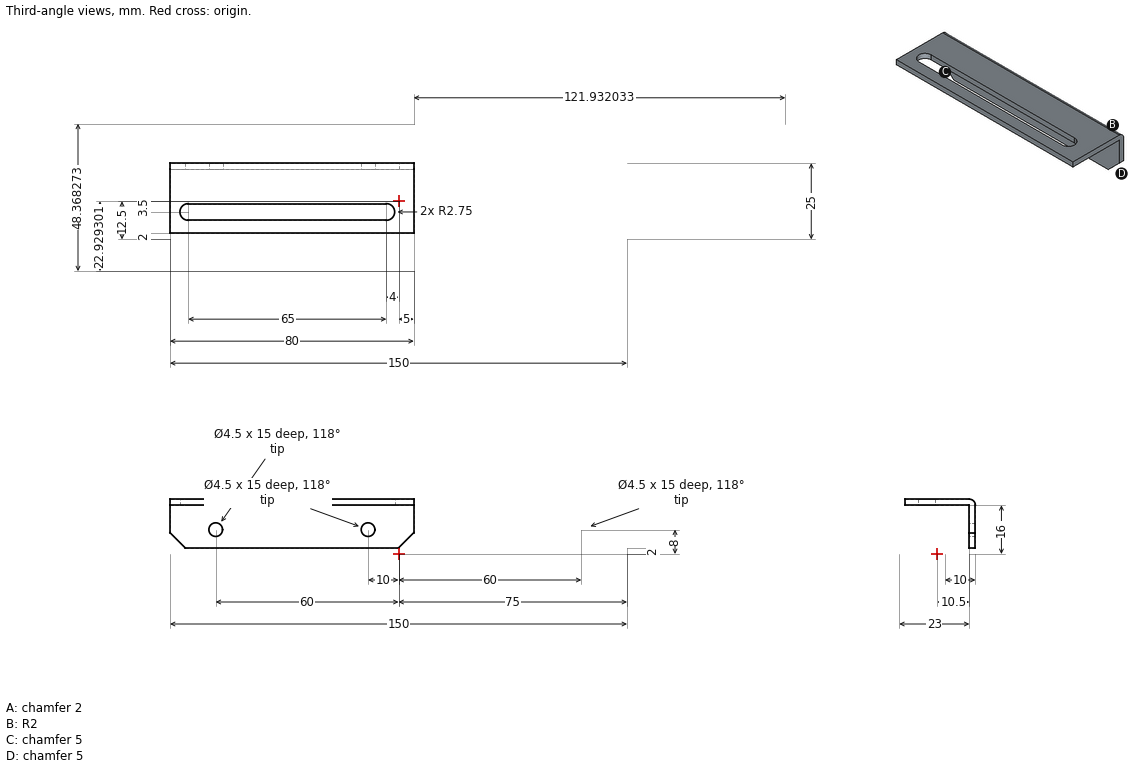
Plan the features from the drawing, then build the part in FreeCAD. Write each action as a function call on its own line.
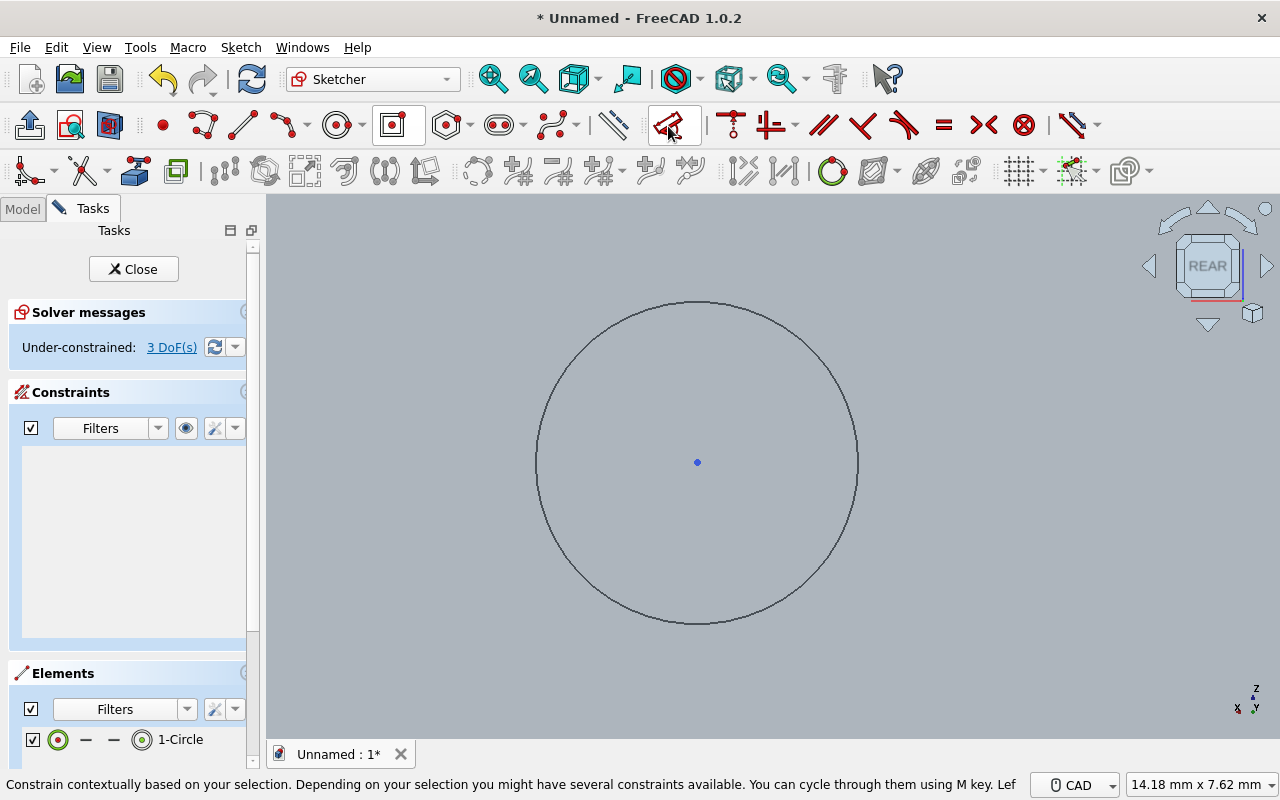
click(811, 349)
click(834, 326)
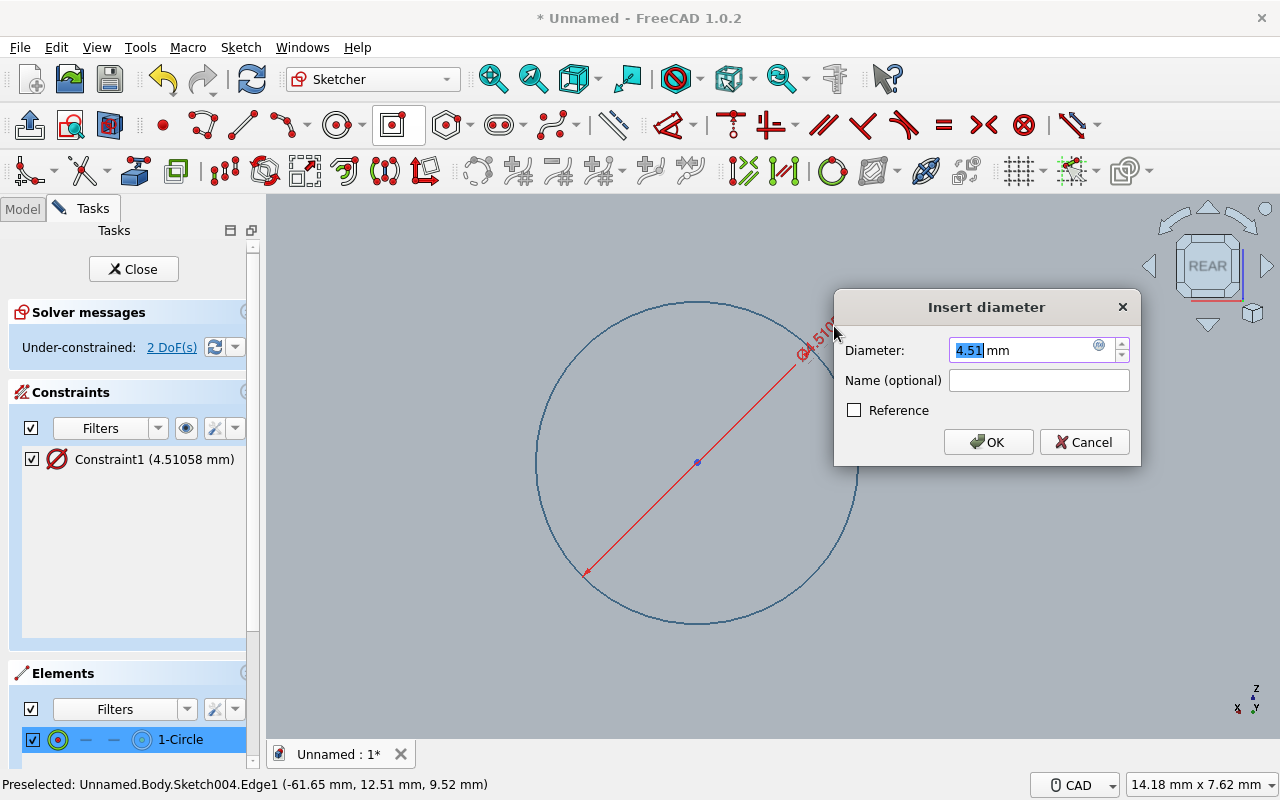
text(4.5)
key(Return)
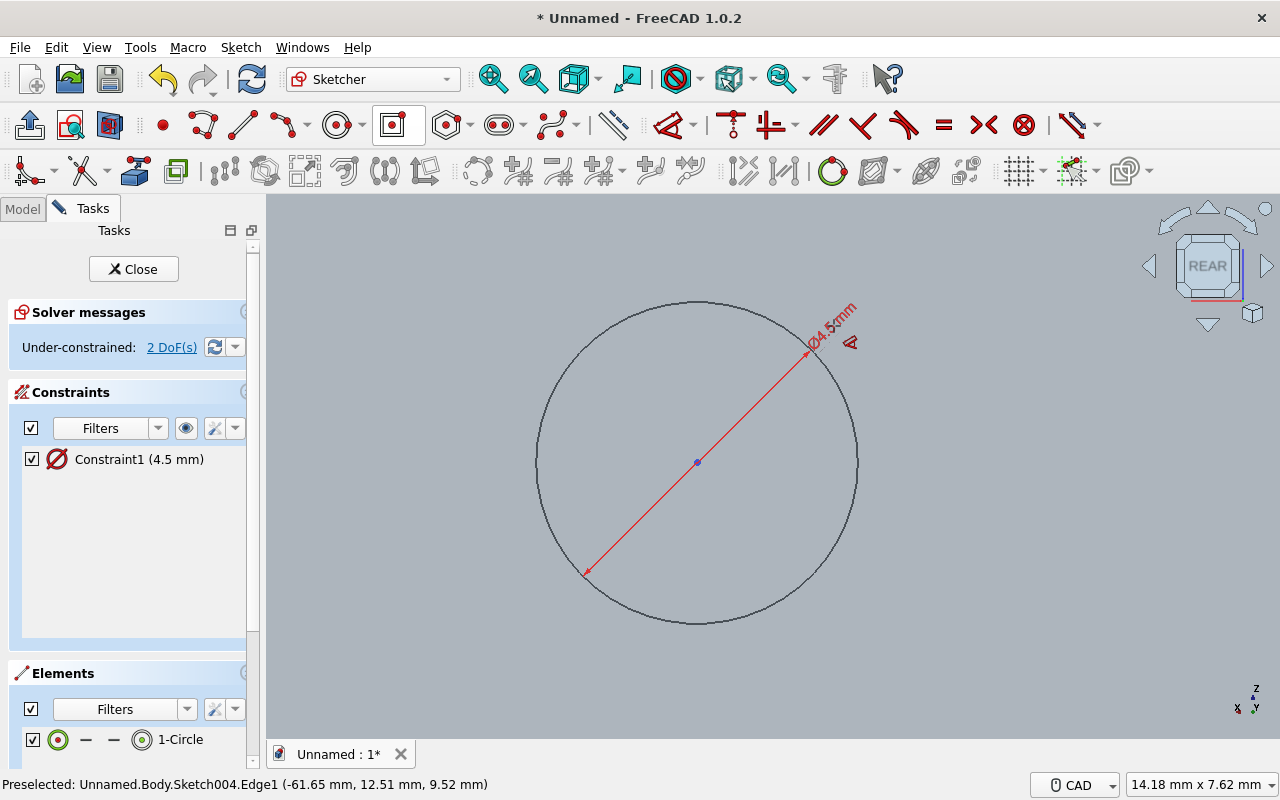
click(697, 463)
click(731, 587)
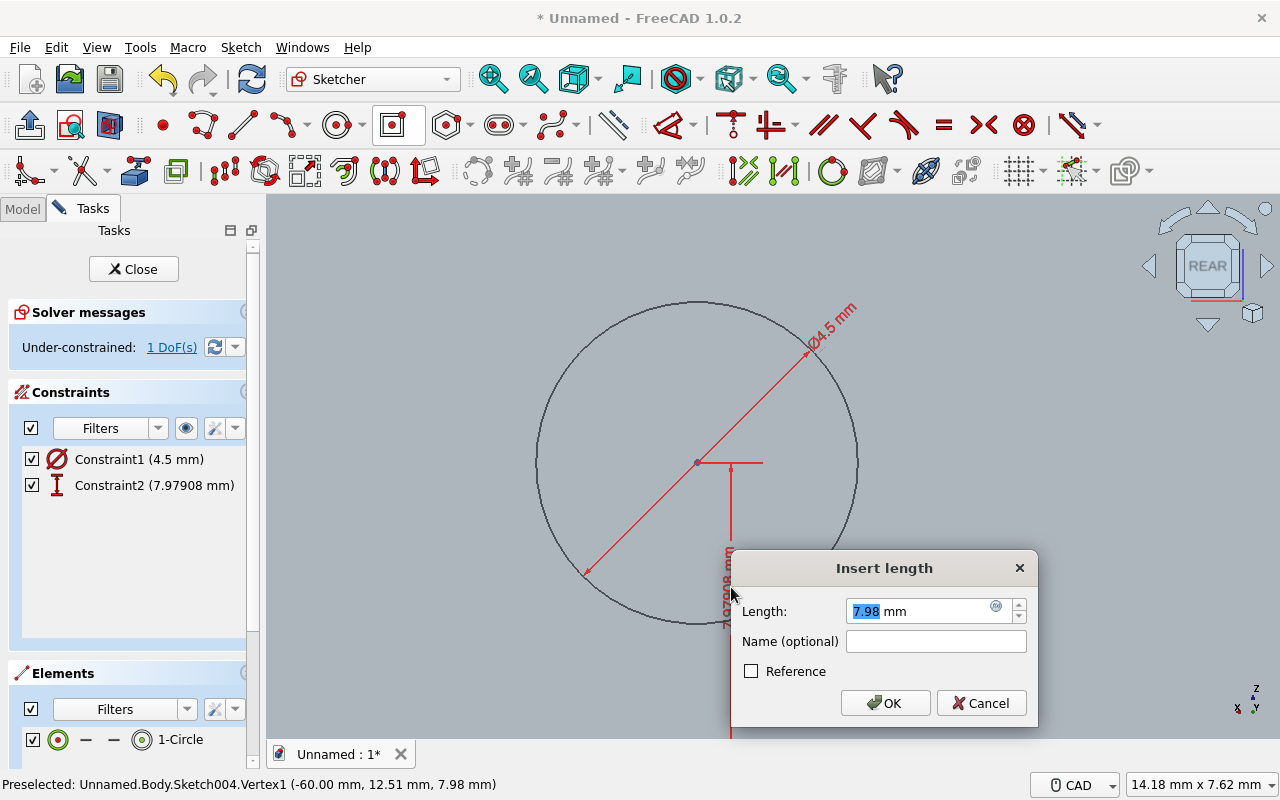
text(8)
key(Return)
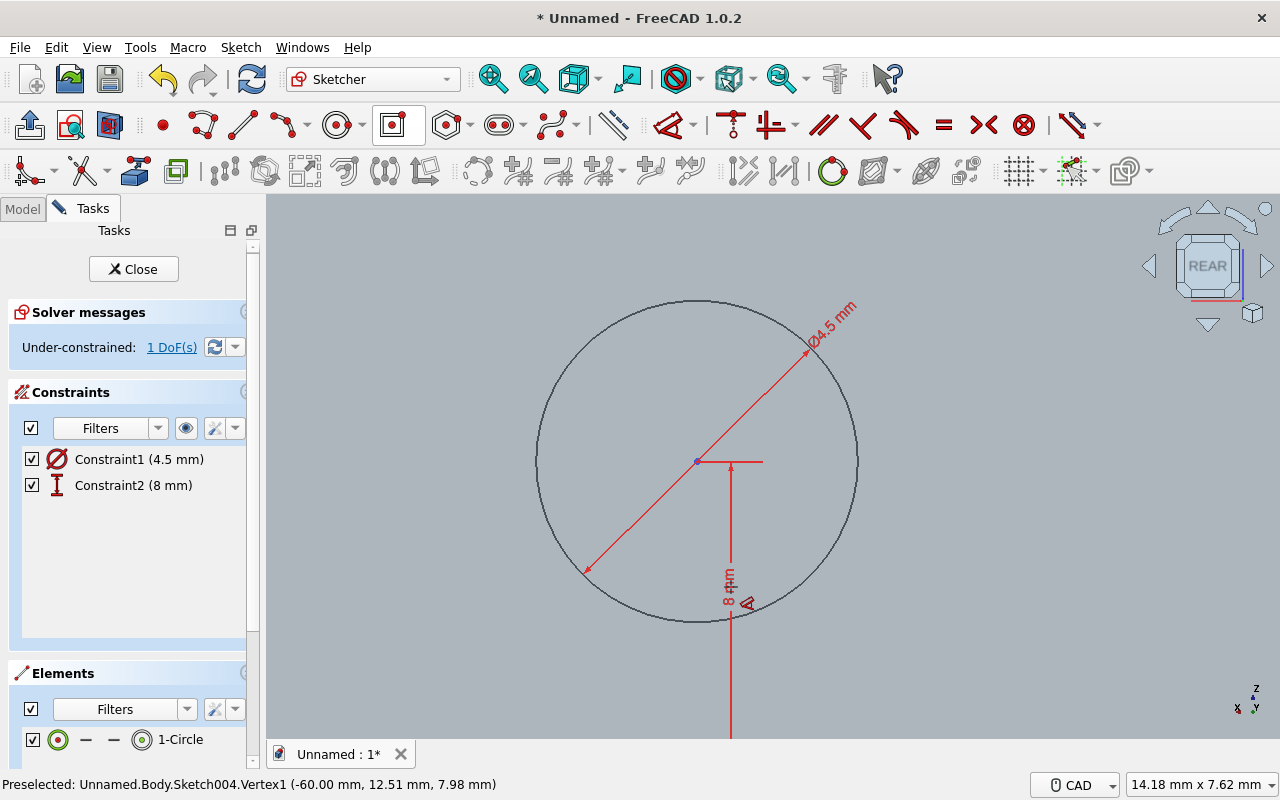
click(697, 462)
click(496, 428)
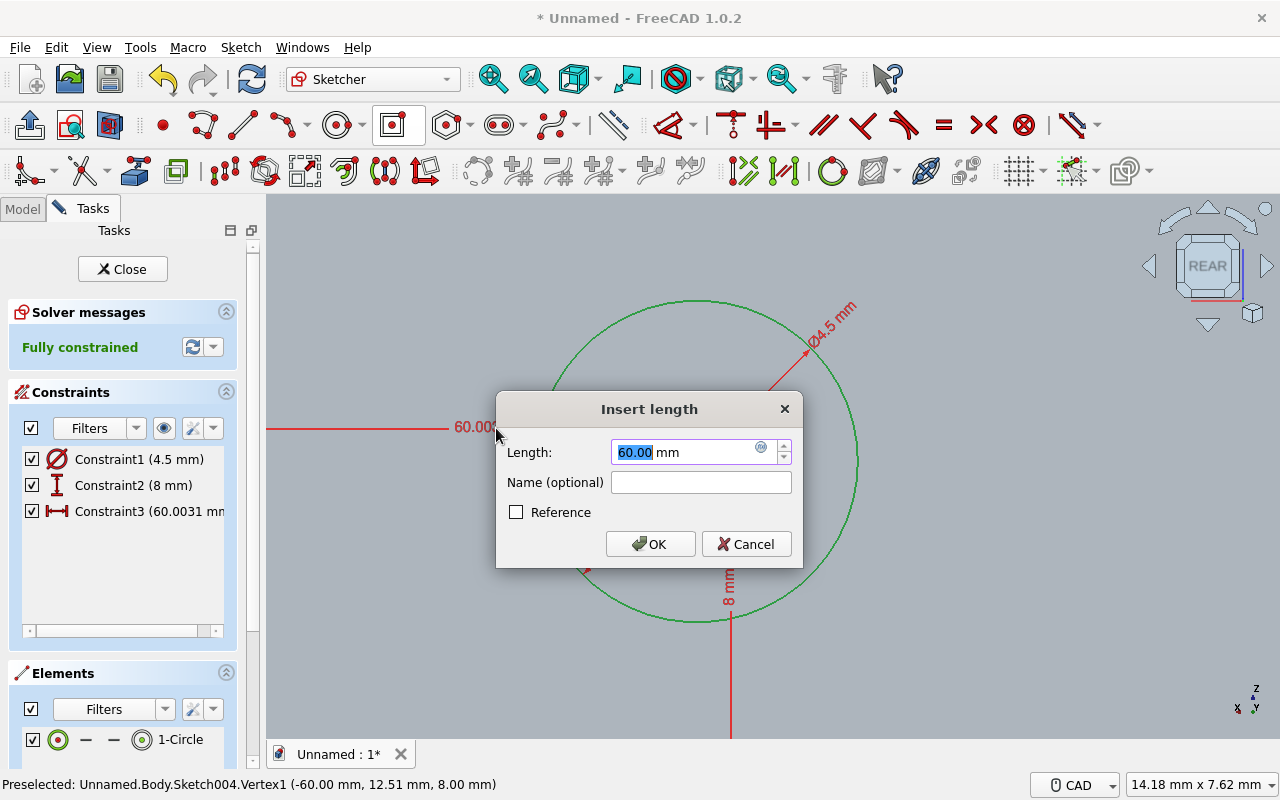
text(60)
key(Return)
key(Escape)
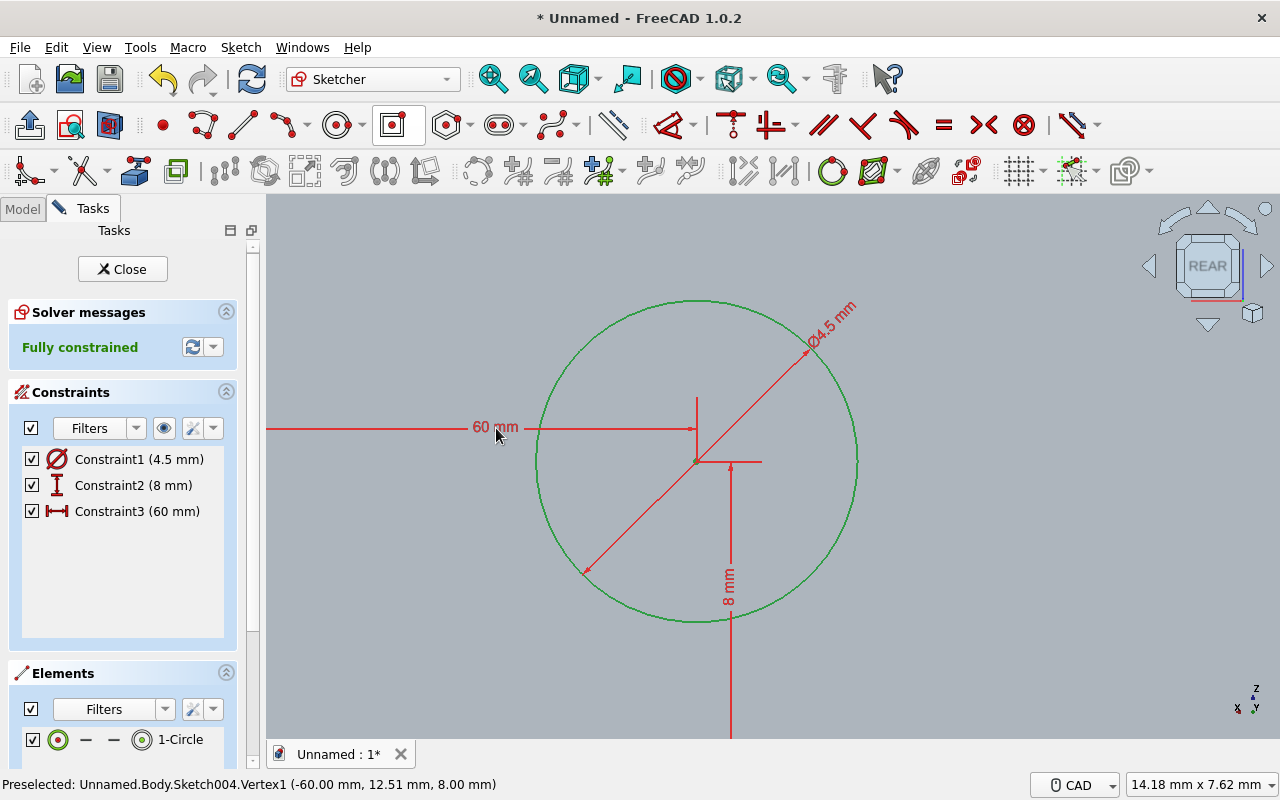
click(123, 269)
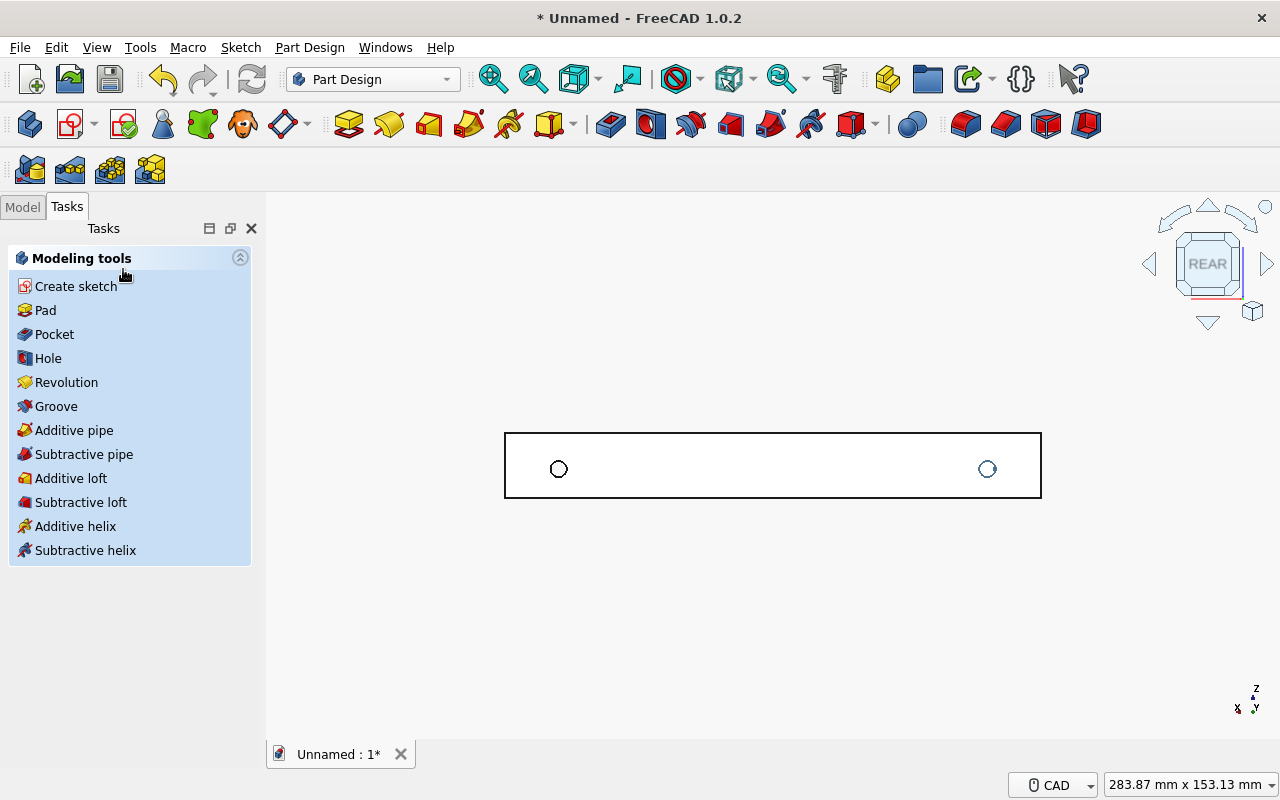
click(652, 124)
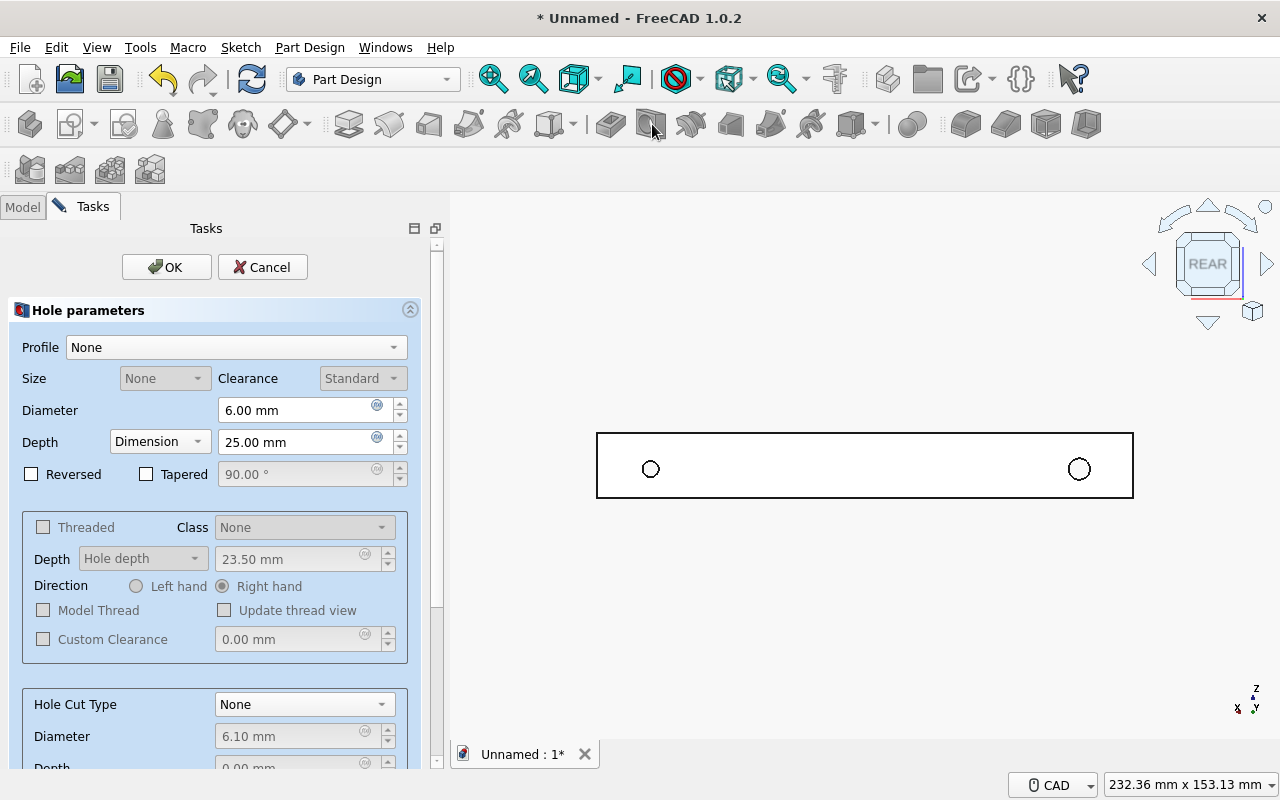
triple_click(305, 410)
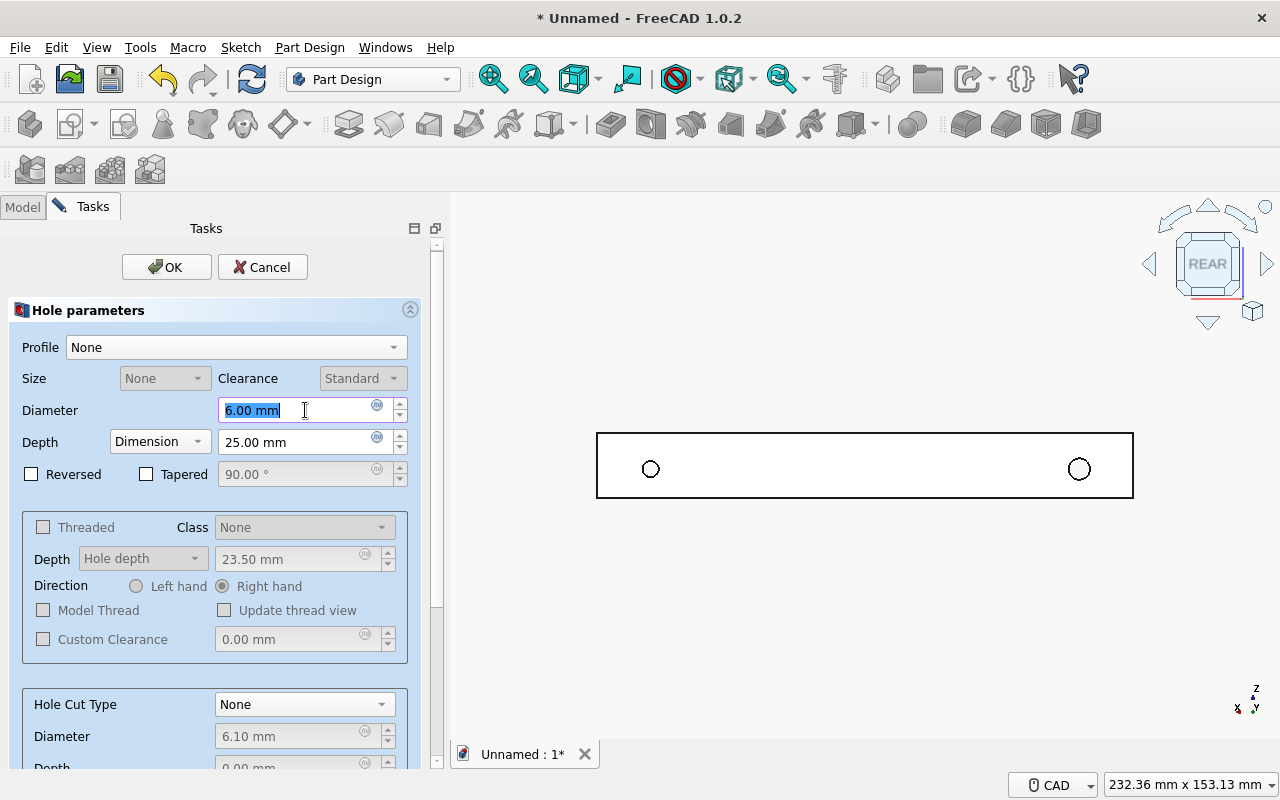
text(4.5)
key(Tab)